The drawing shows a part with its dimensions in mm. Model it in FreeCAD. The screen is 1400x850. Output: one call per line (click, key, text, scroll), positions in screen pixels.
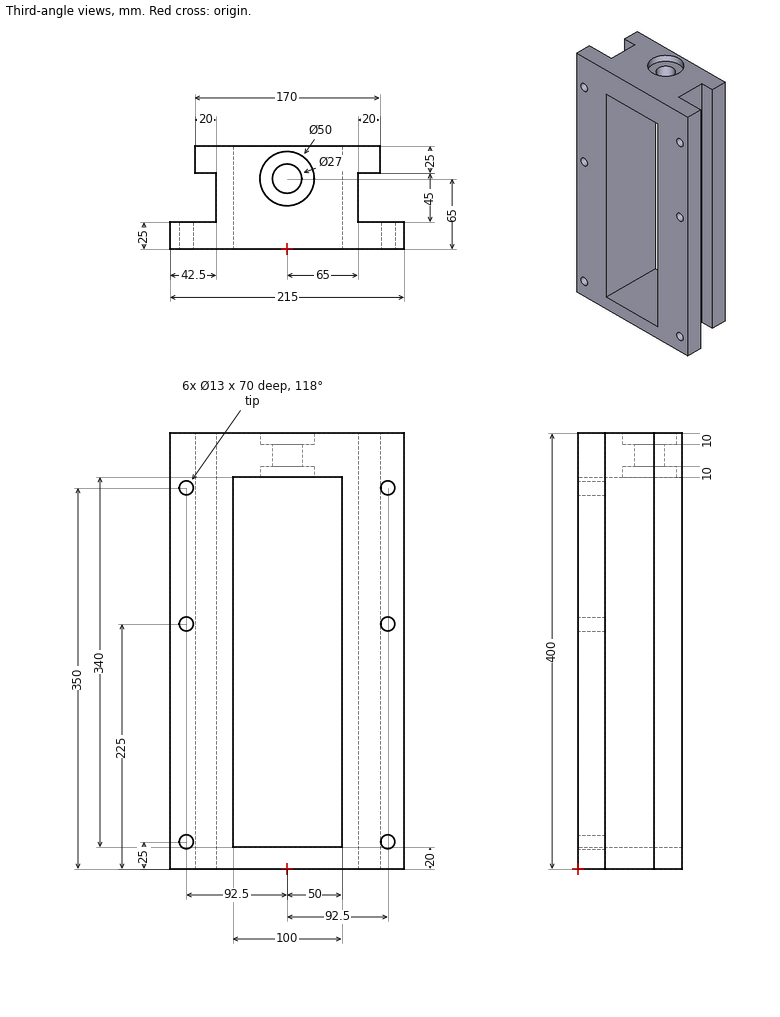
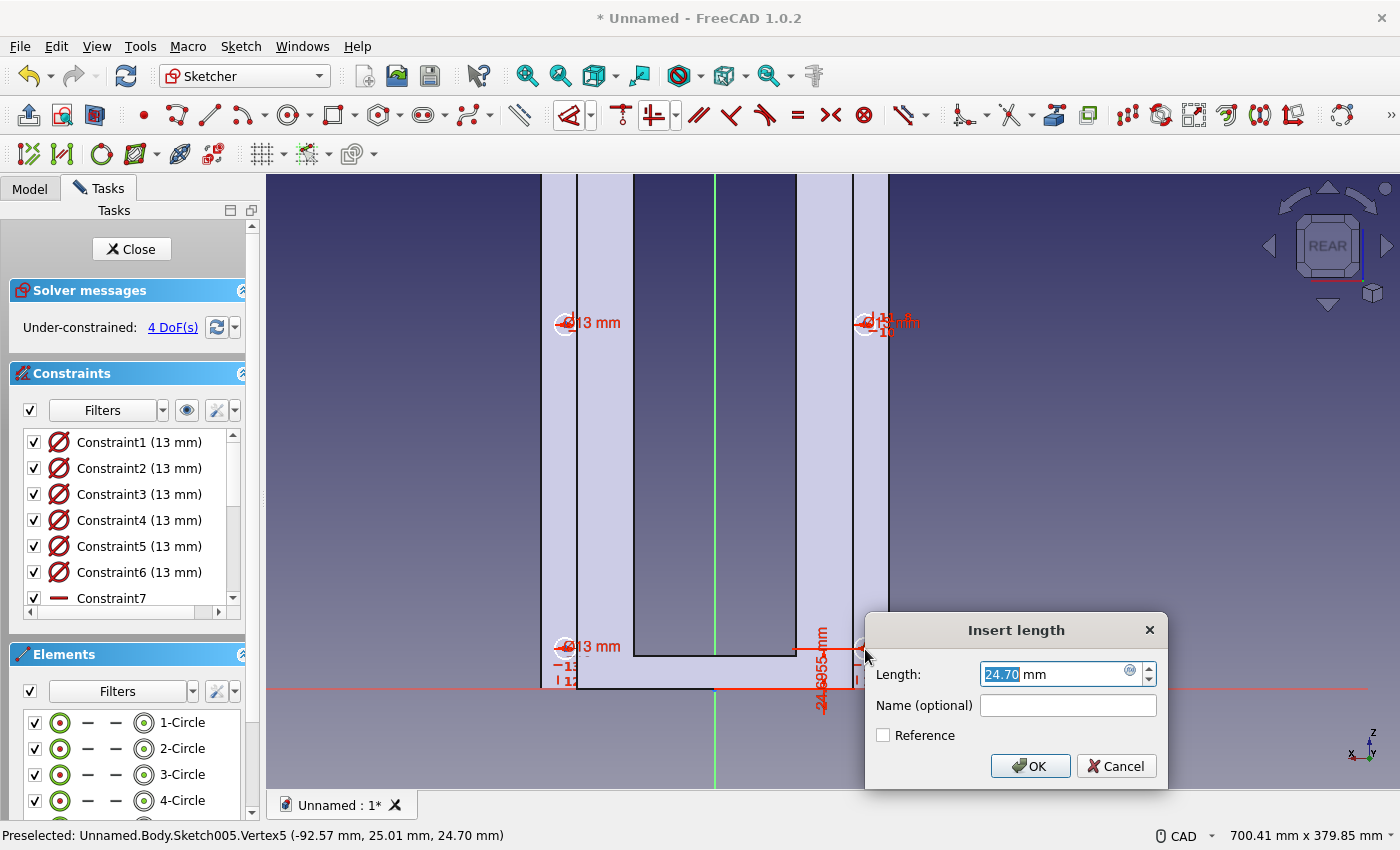
text(25)
key(Return)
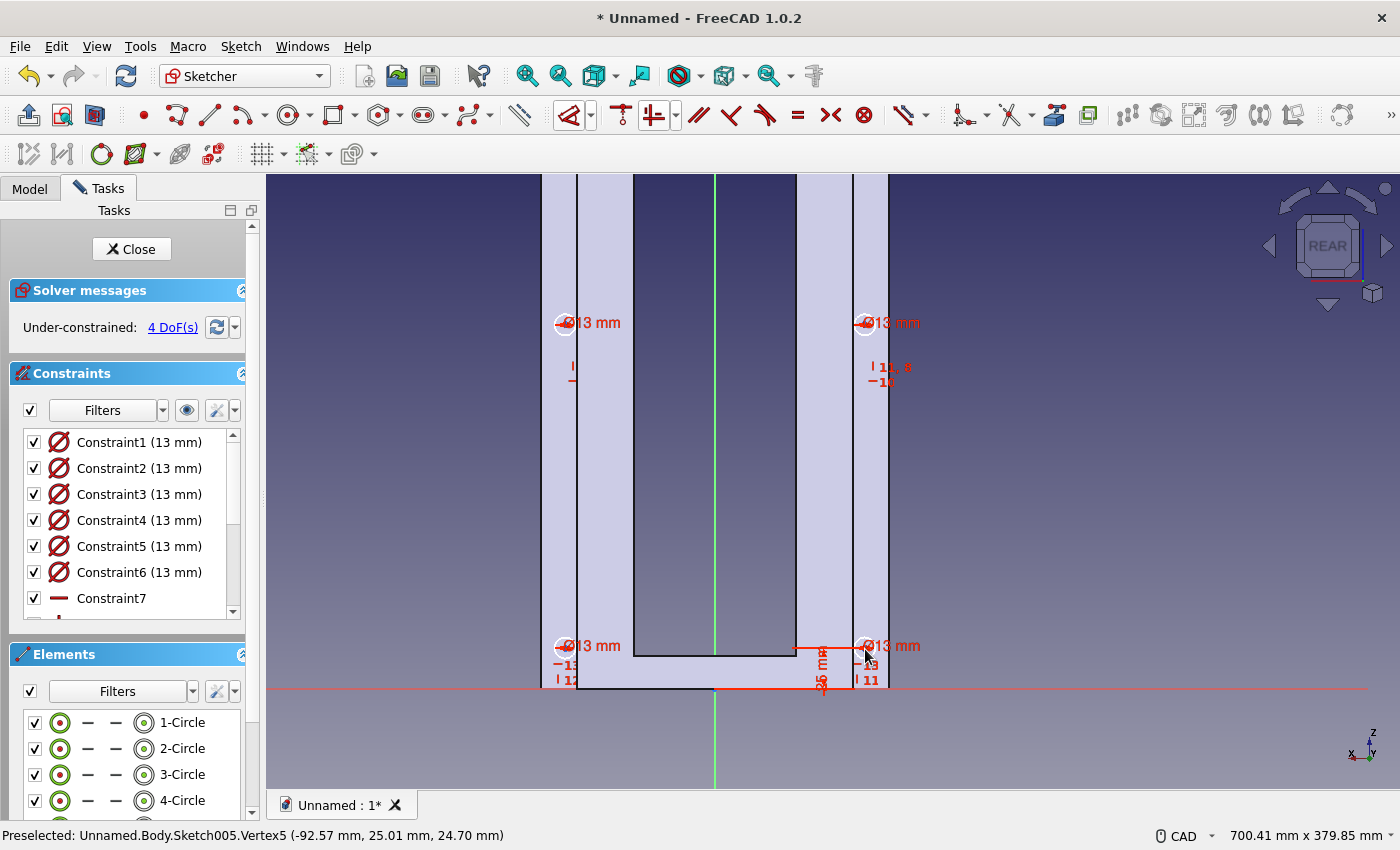
scroll(865, 647, down, 2)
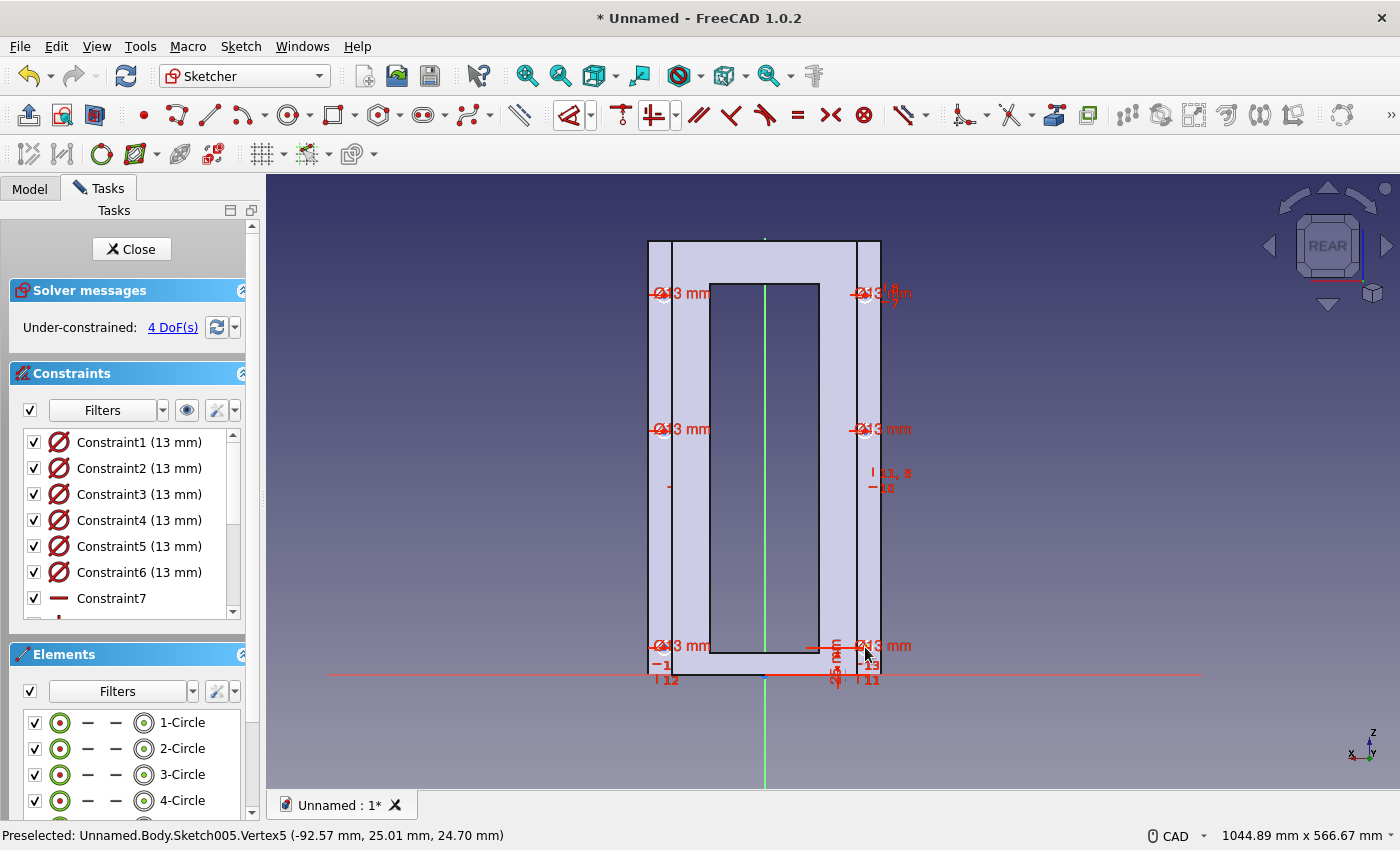
click(865, 295)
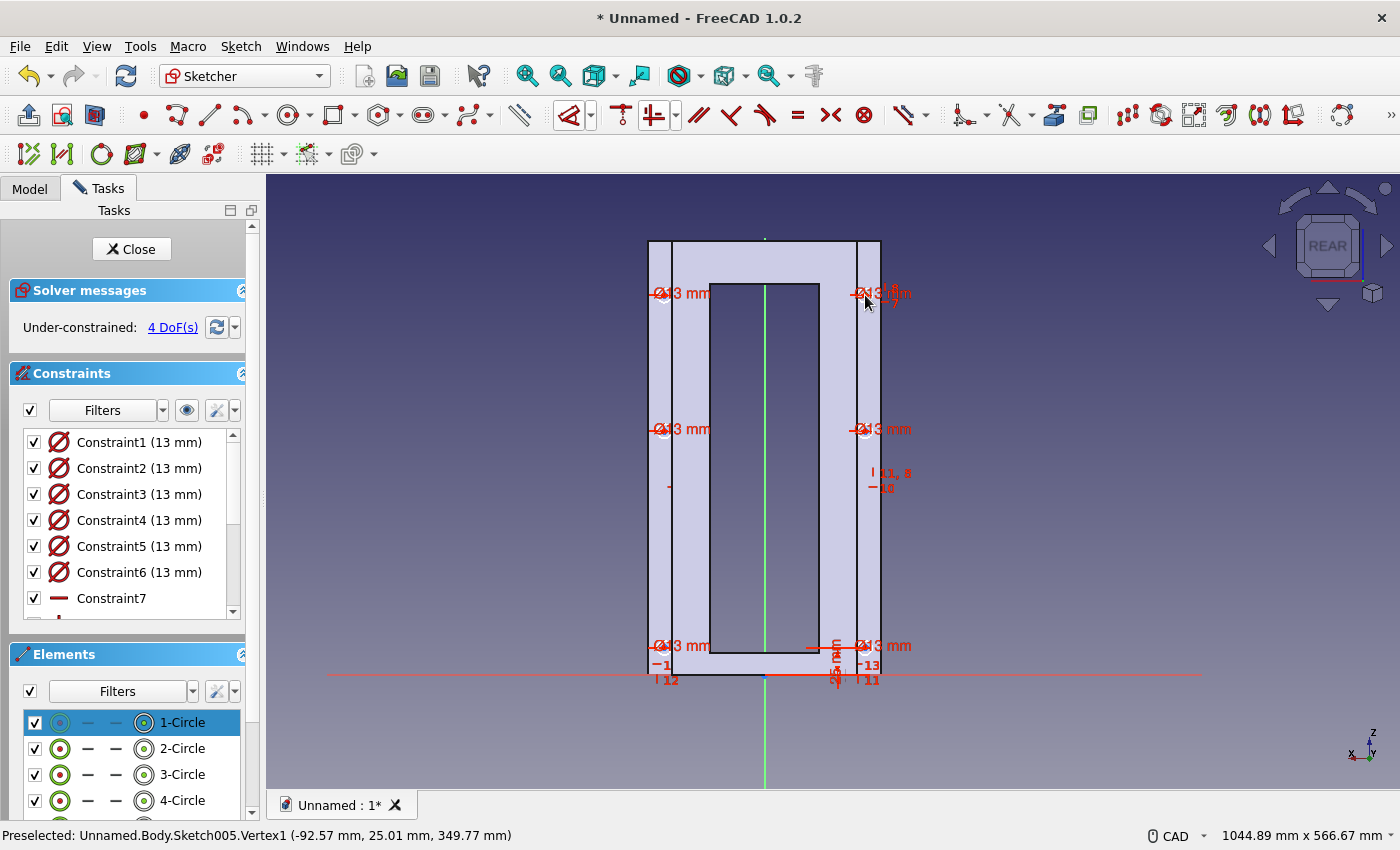
key(i)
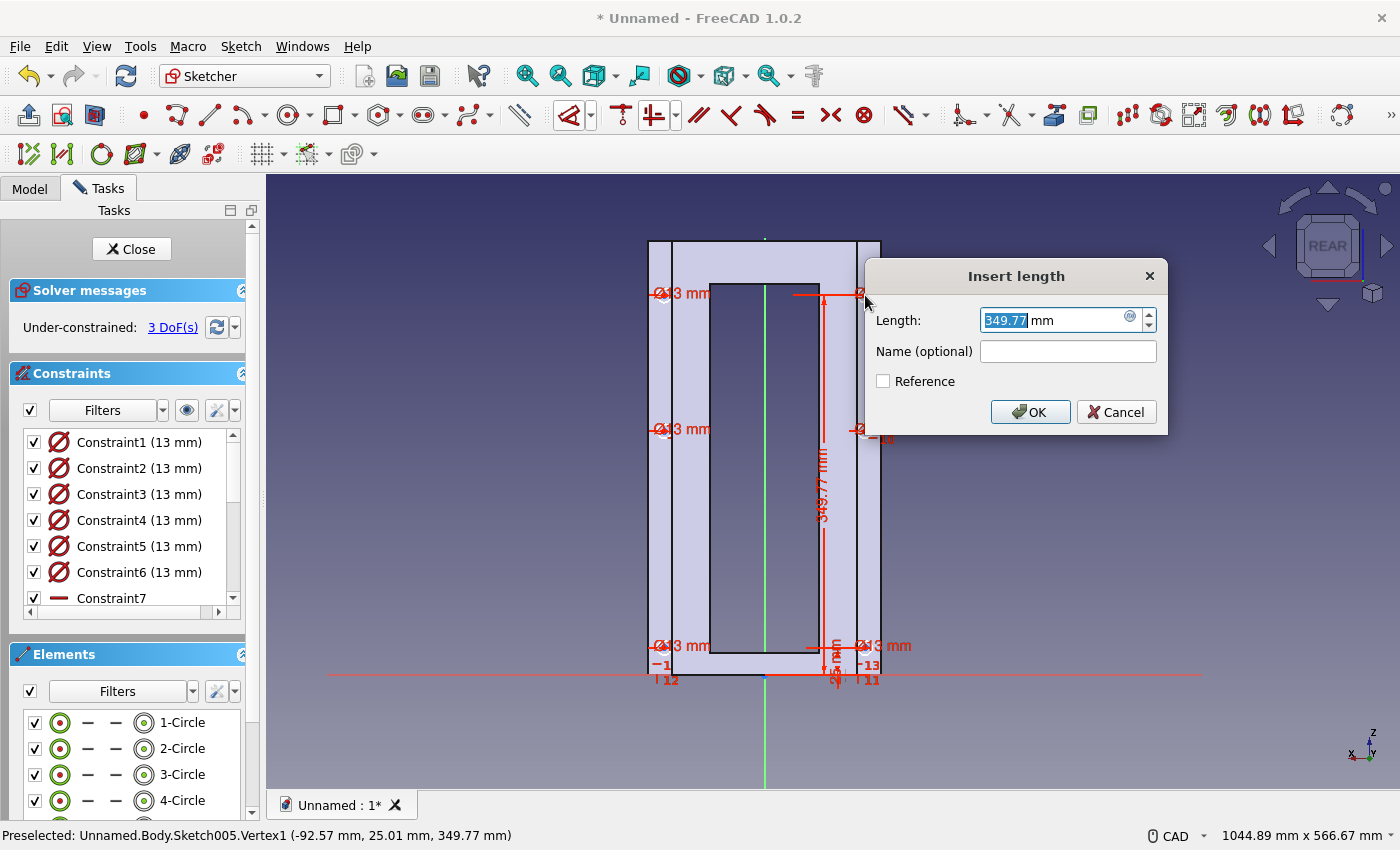
text(350)
key(Return)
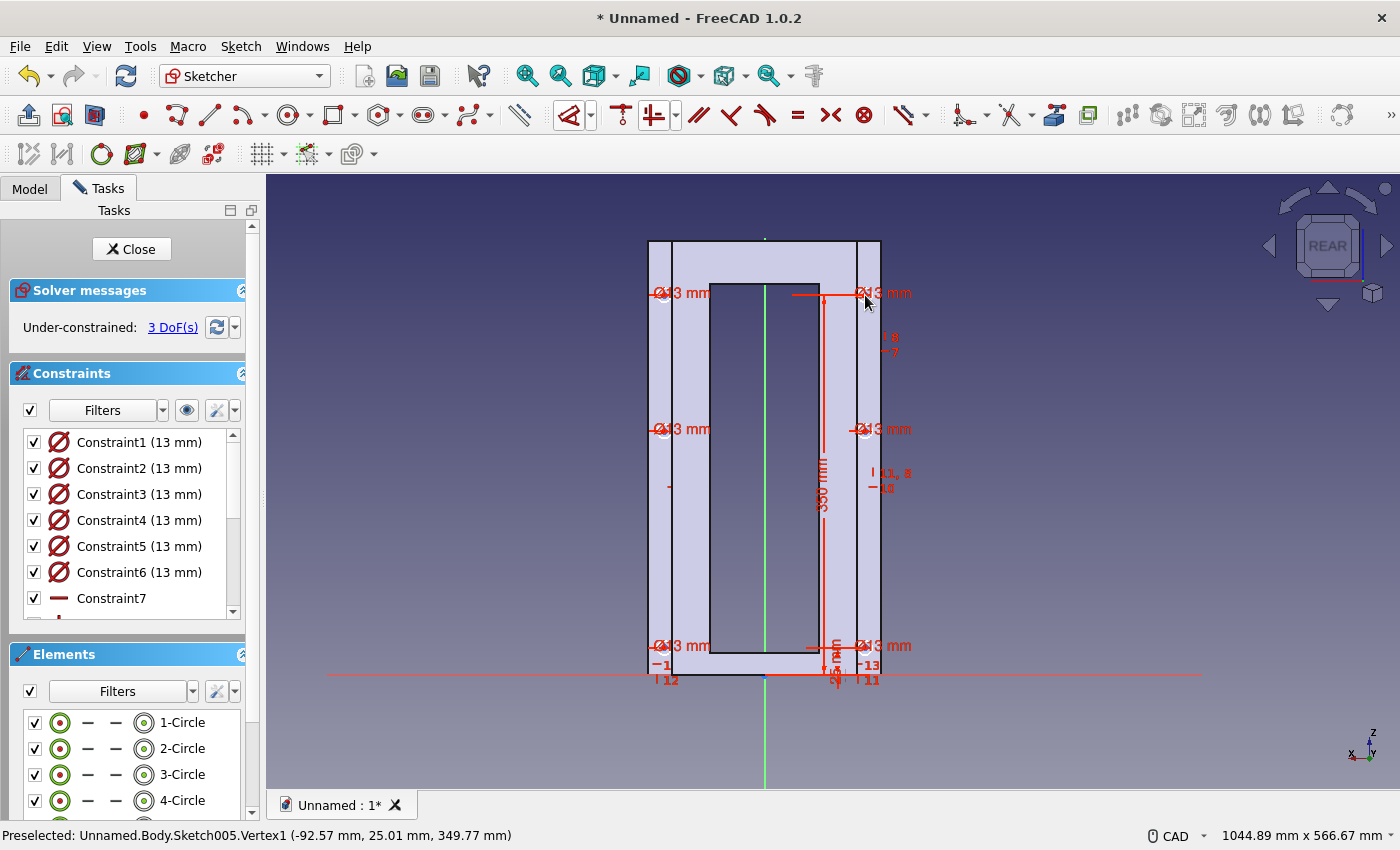
click(865, 431)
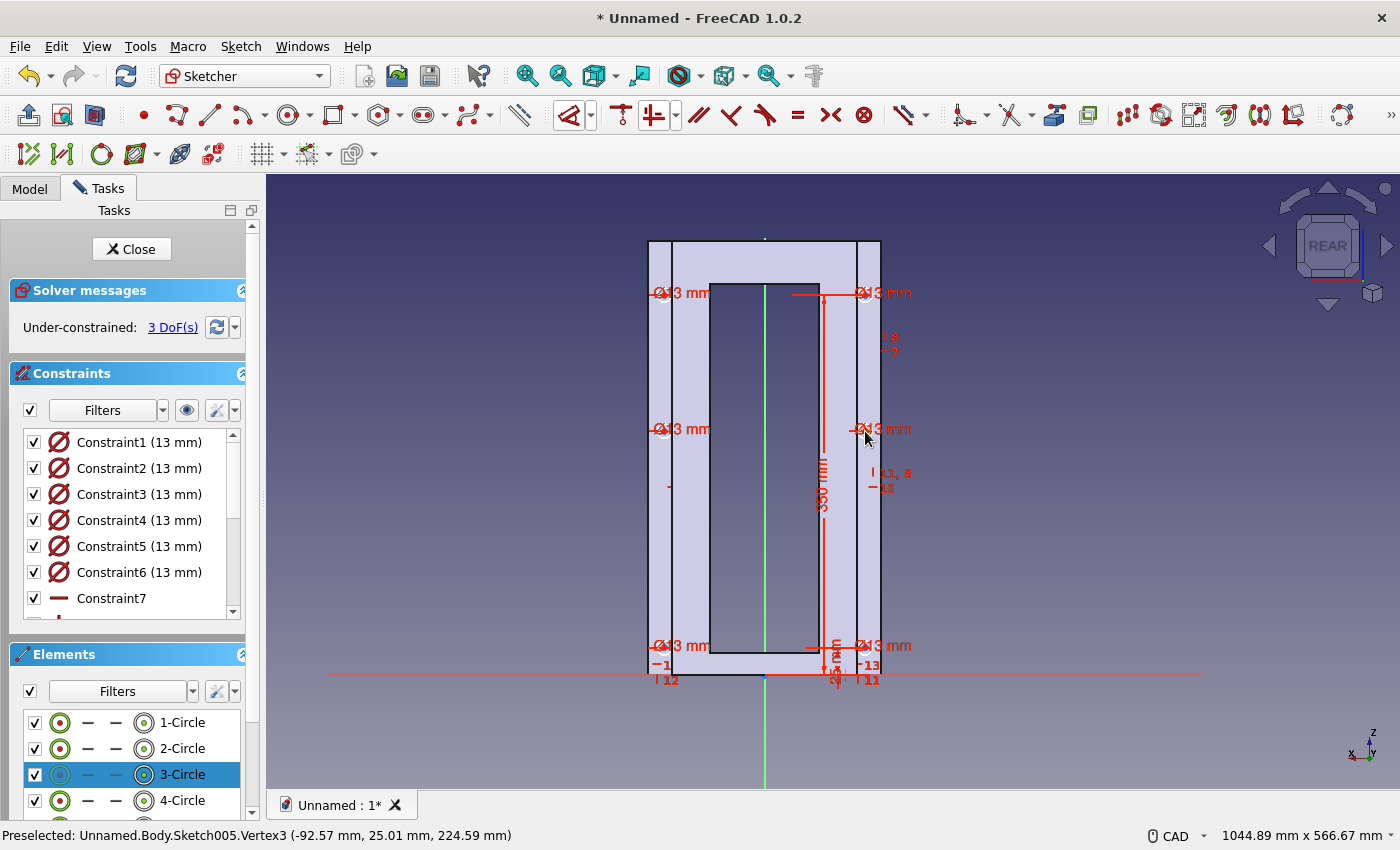
key(i)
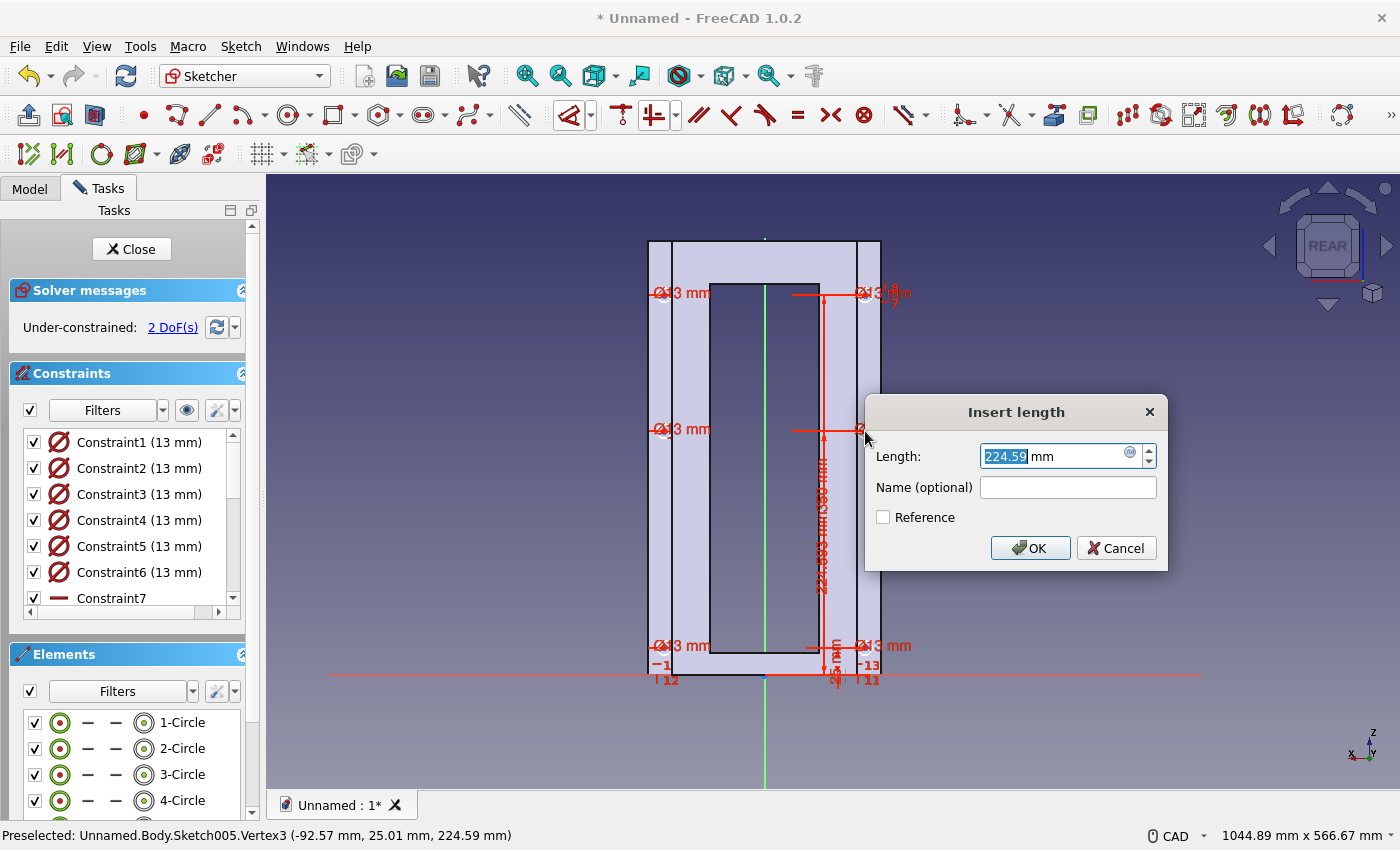
text(225)
key(Return)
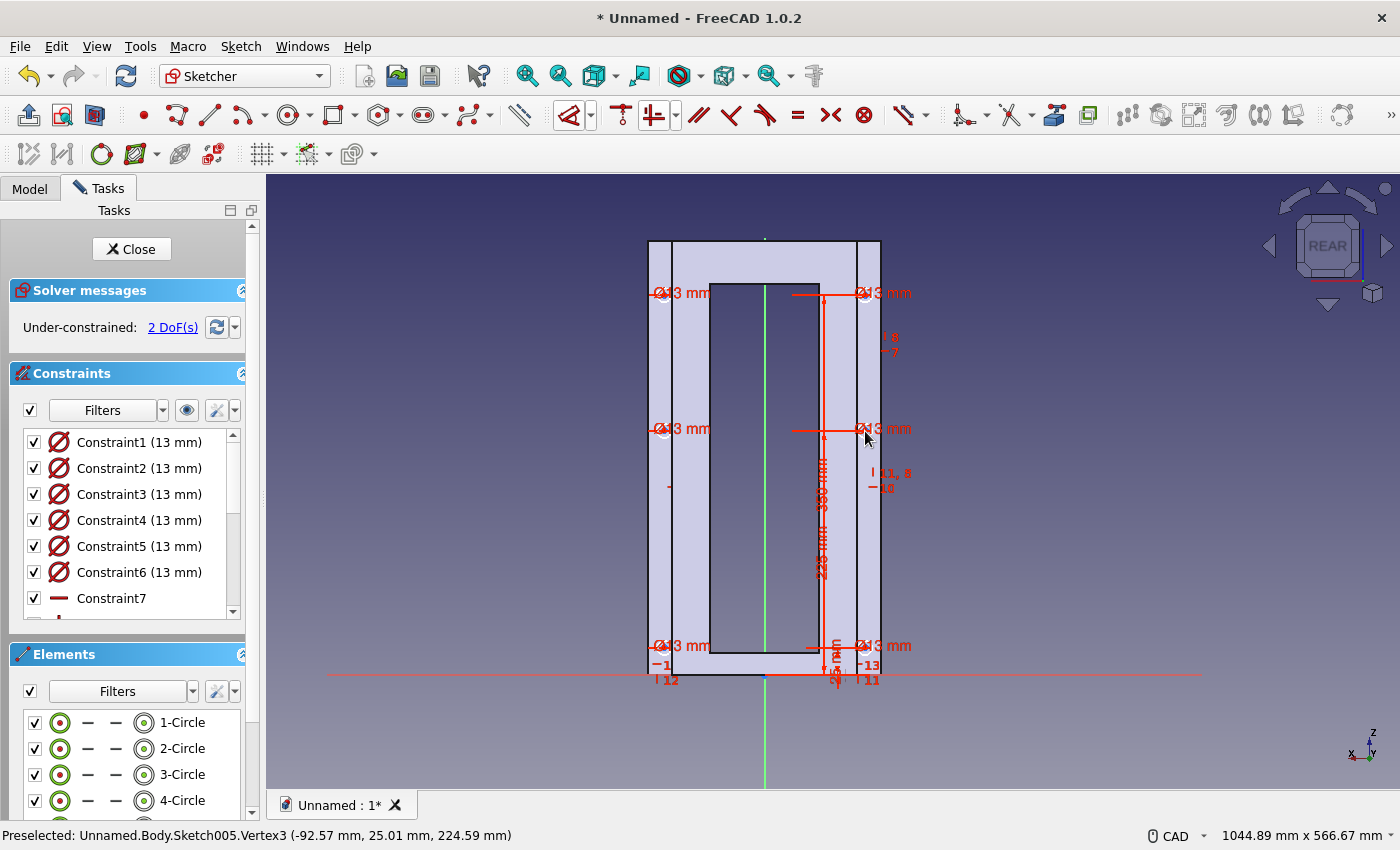
click(865, 295)